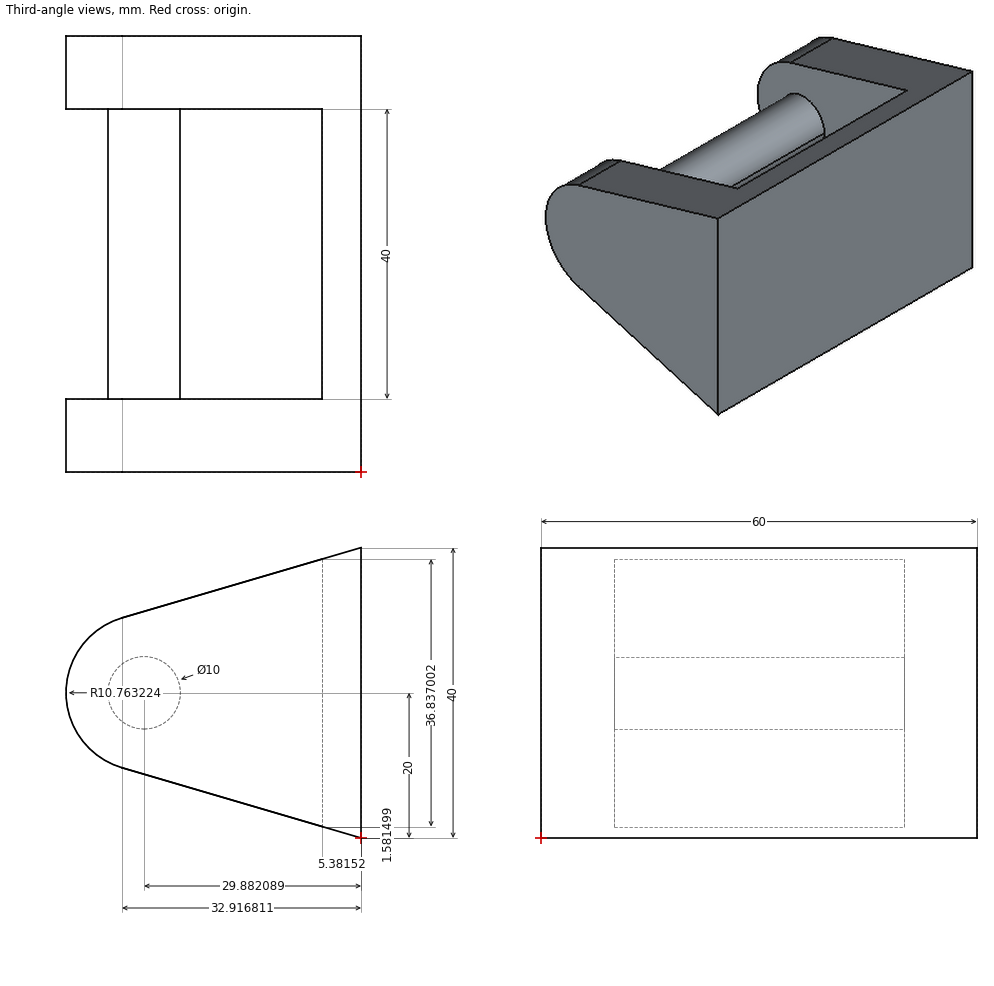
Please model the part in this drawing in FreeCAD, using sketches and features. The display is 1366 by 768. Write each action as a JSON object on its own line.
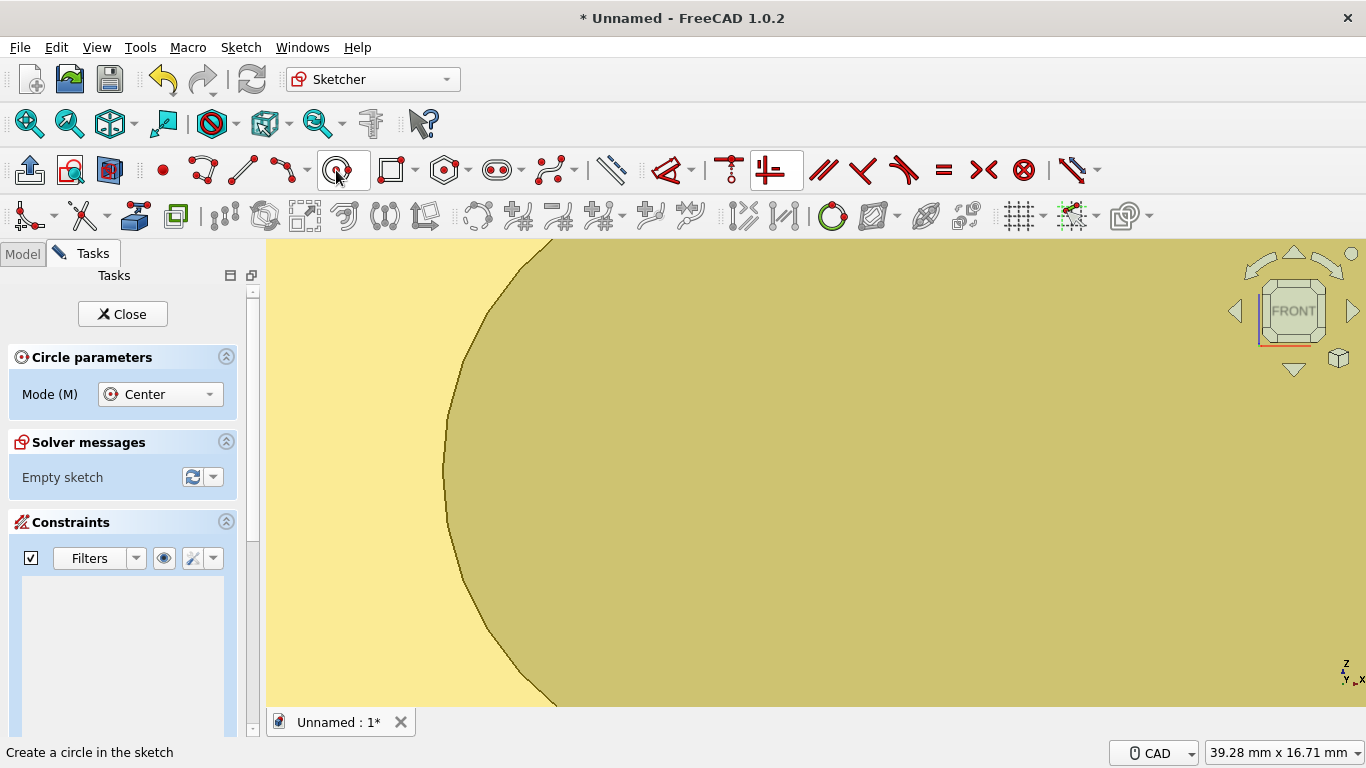
{"action": "left_click", "coordinate": [744, 471]}
{"action": "left_click", "coordinate": [843, 372]}
{"action": "key", "text": "Escape"}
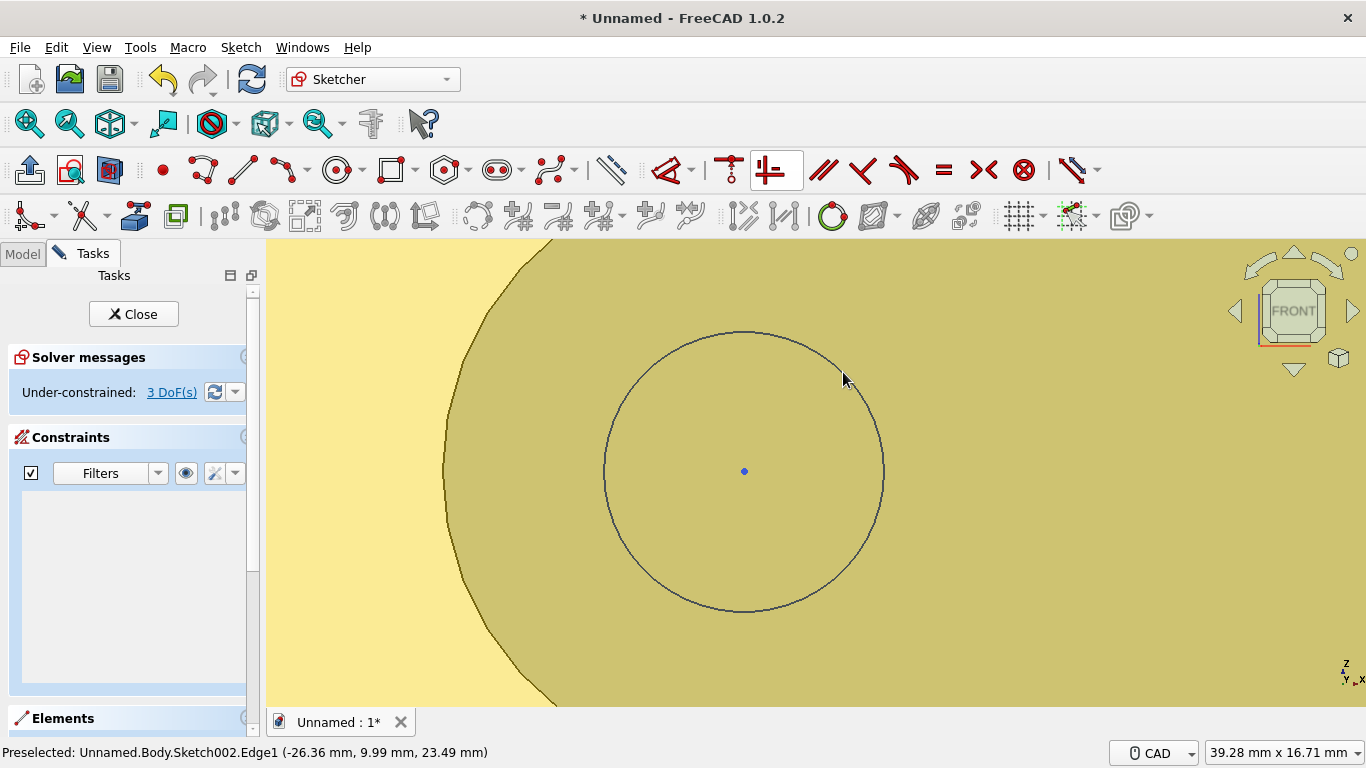
{"action": "left_click", "coordinate": [666, 170]}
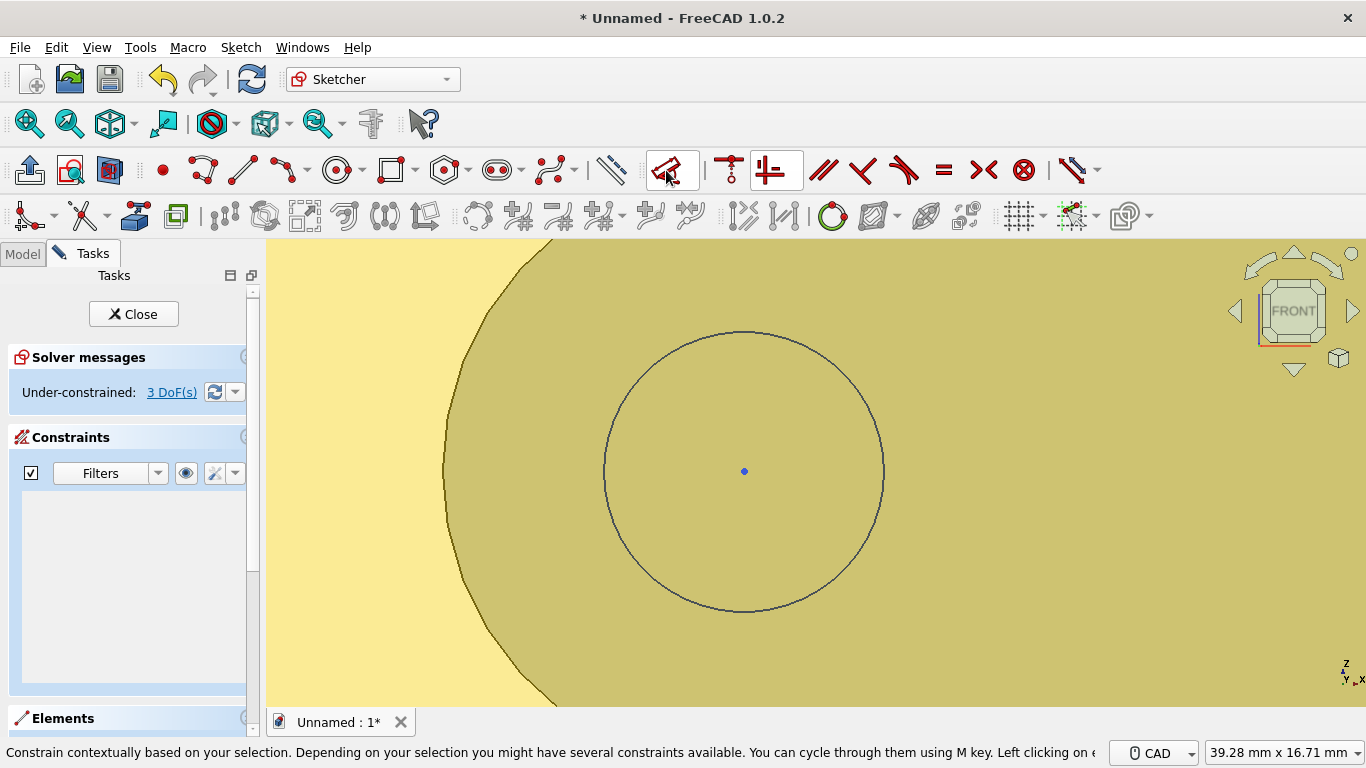
{"action": "left_click", "coordinate": [843, 373]}
{"action": "left_click", "coordinate": [866, 350]}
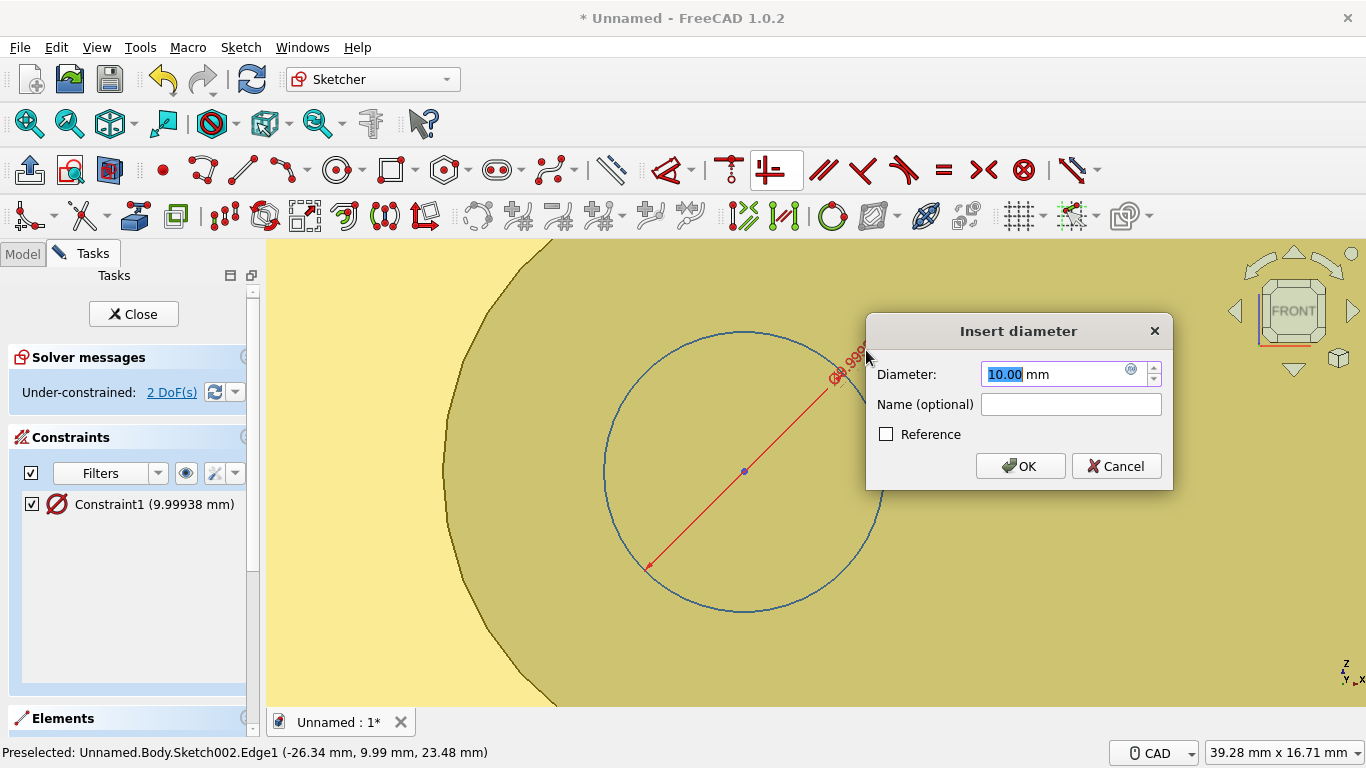
{"action": "type", "text": "10"}
{"action": "key", "text": "Return"}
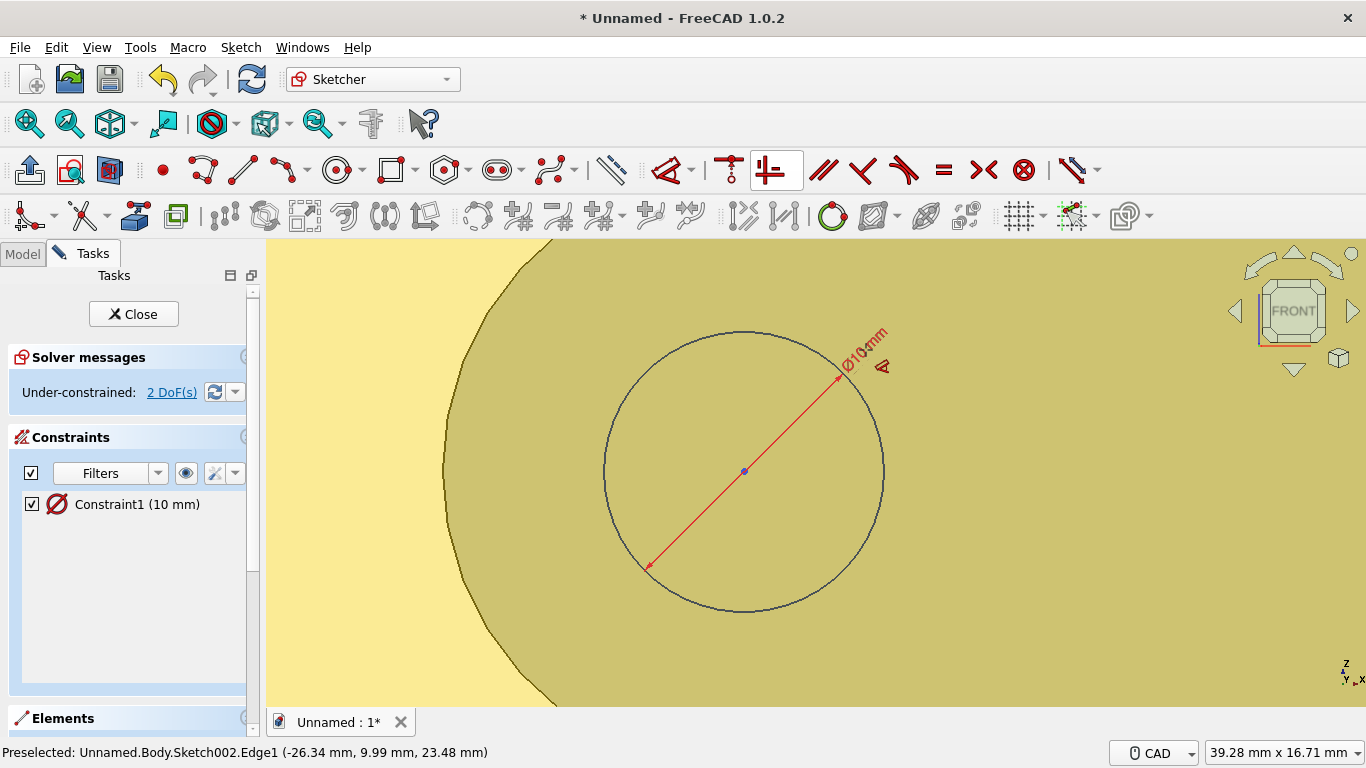
{"action": "left_click", "coordinate": [744, 472]}
{"action": "left_click", "coordinate": [710, 575]}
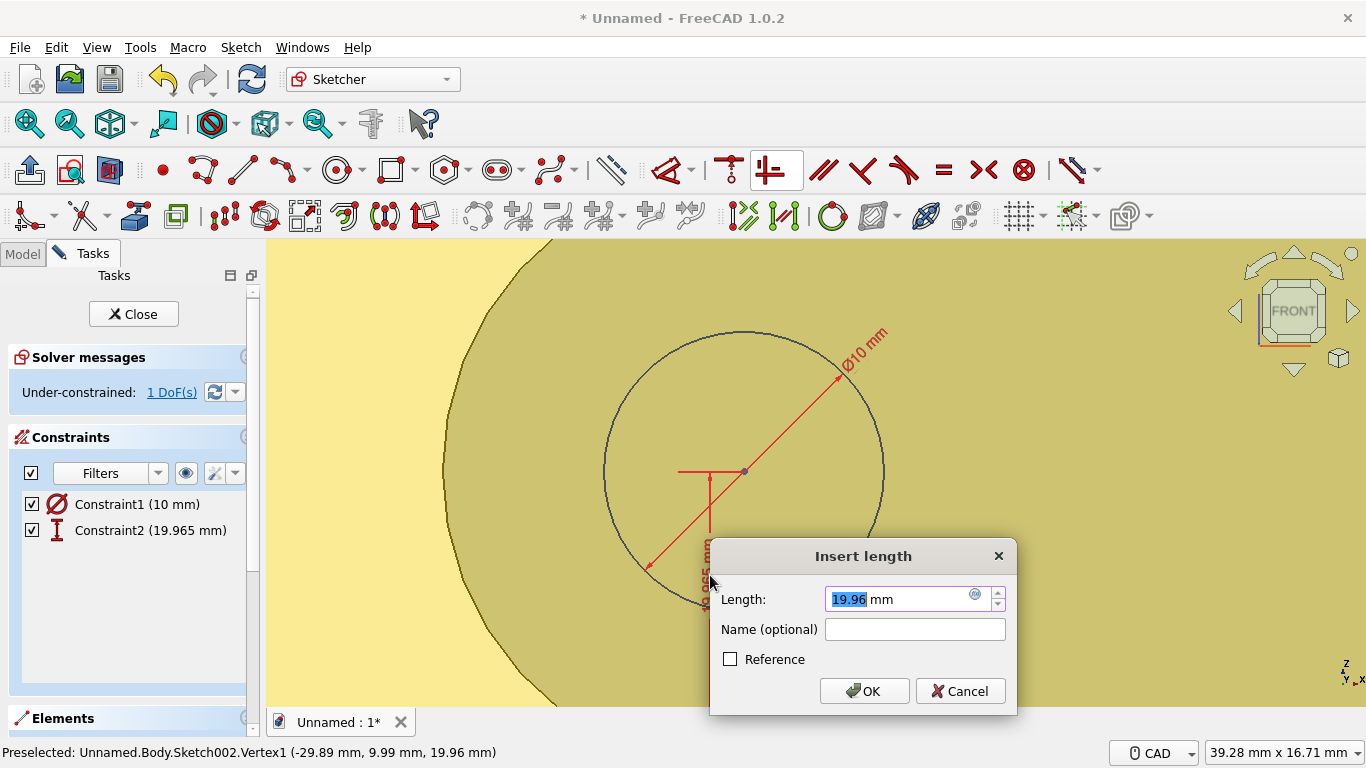
{"action": "type", "text": "20"}
{"action": "key", "text": "Return"}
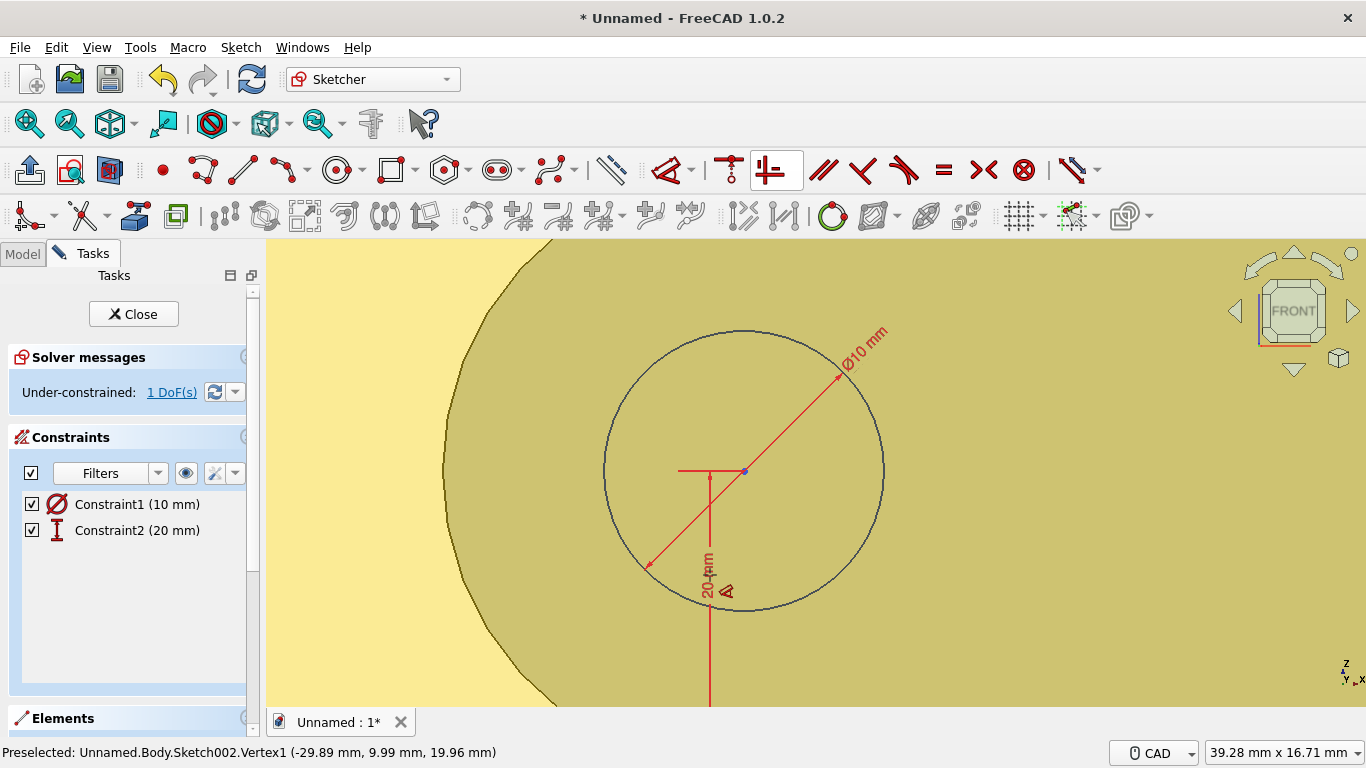
{"action": "left_click", "coordinate": [744, 471]}
{"action": "left_click", "coordinate": [973, 437]}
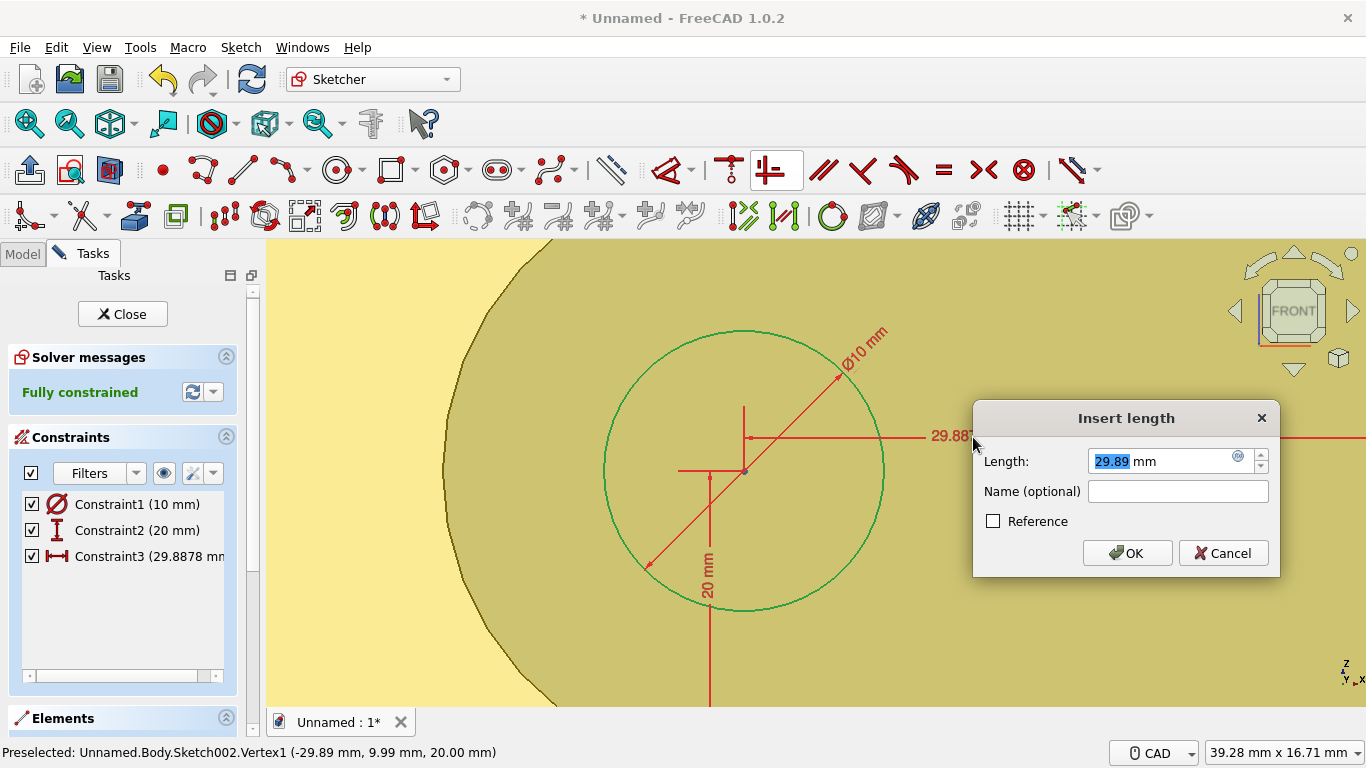
{"action": "type", "text": "29.882089"}
{"action": "key", "text": "Return"}
{"action": "key", "text": "Escape"}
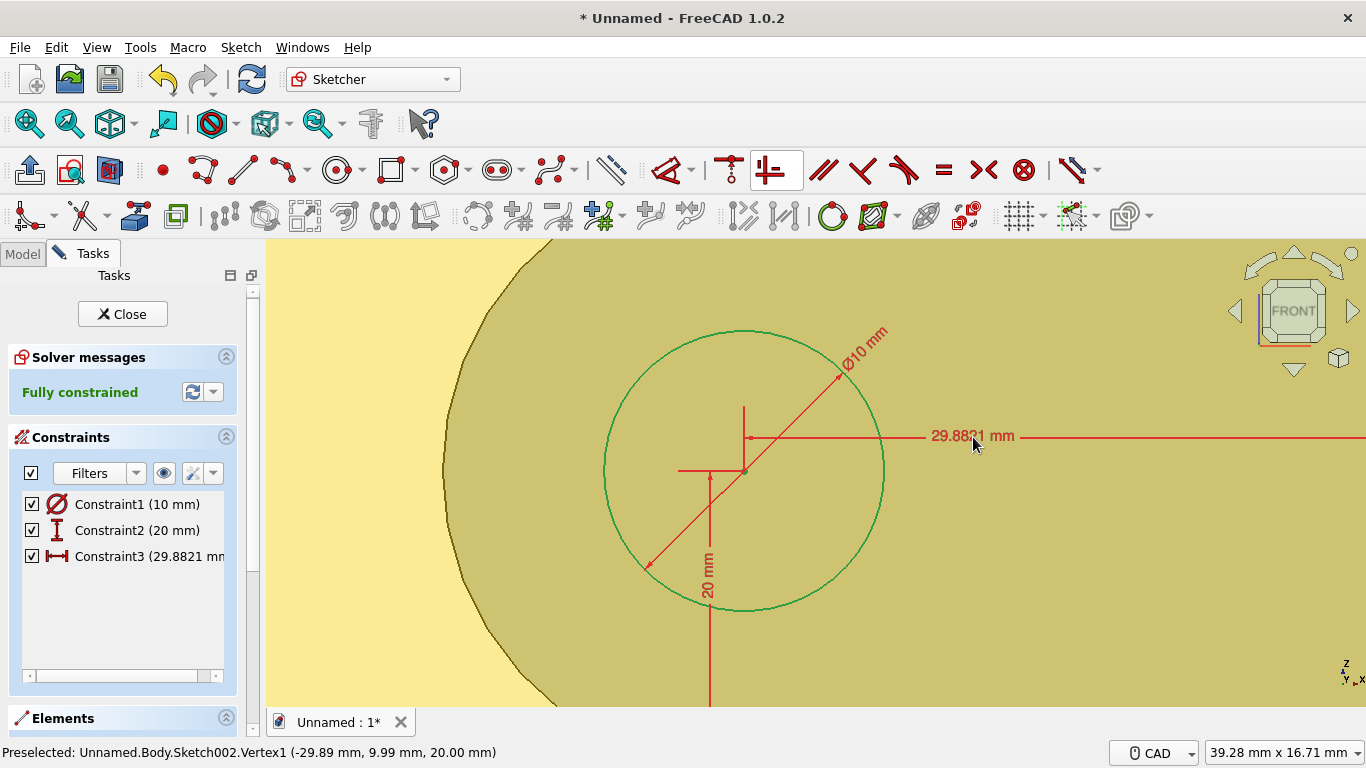
{"action": "left_click", "coordinate": [123, 314]}